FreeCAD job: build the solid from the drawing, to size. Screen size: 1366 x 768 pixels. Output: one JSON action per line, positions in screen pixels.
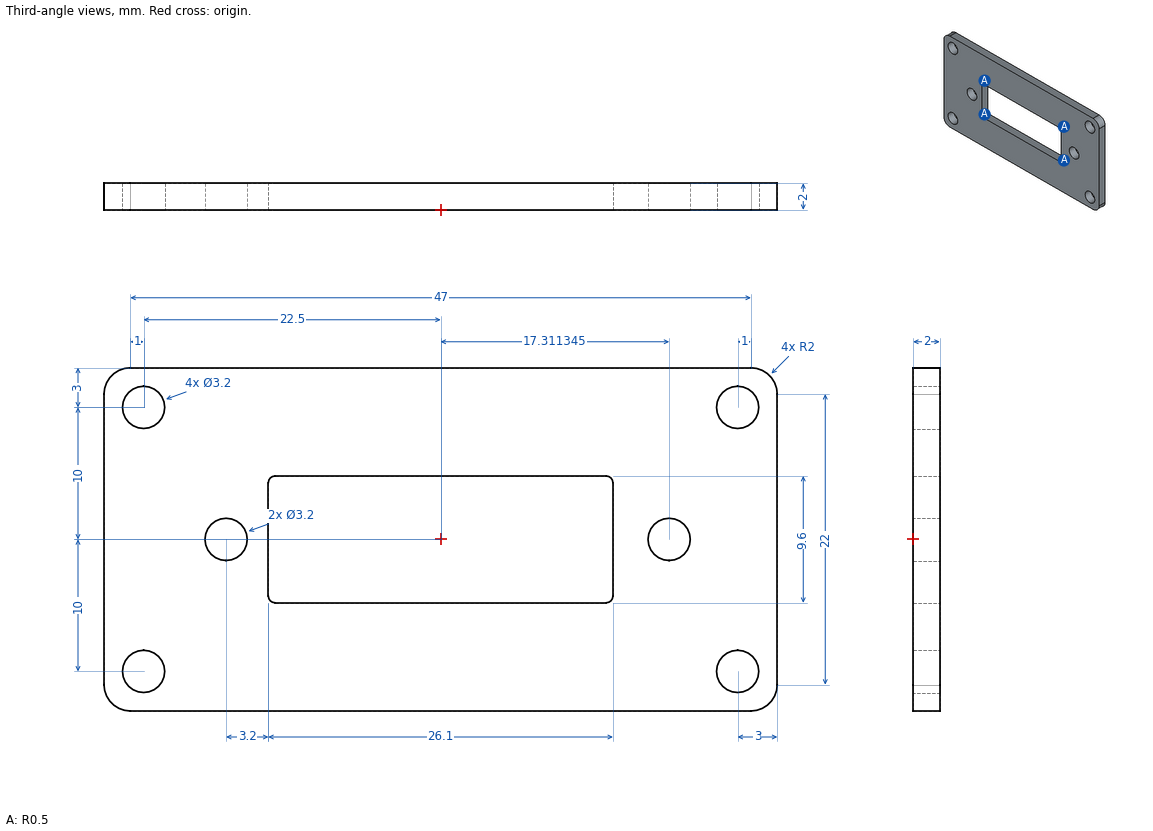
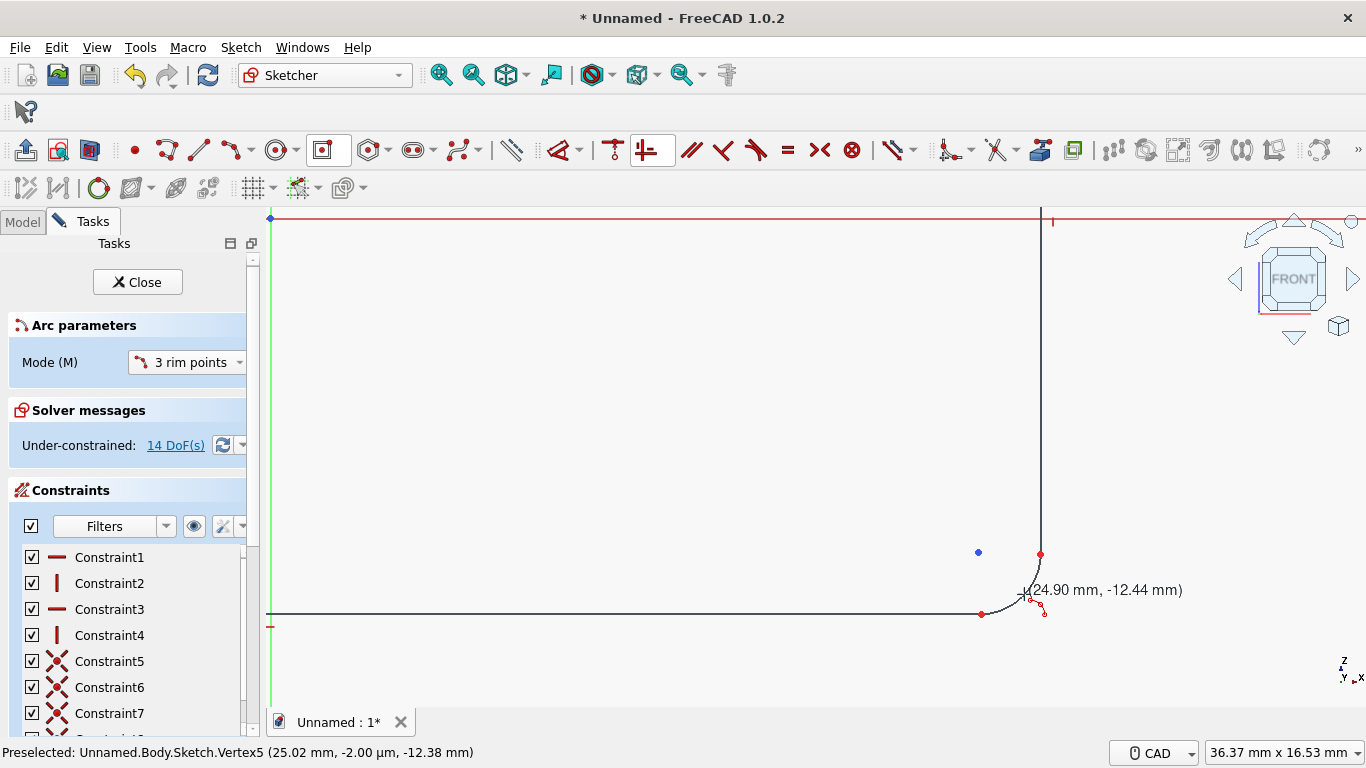
{"action": "scroll", "coordinate": [1025, 596], "scroll_direction": "down", "scroll_amount": 5}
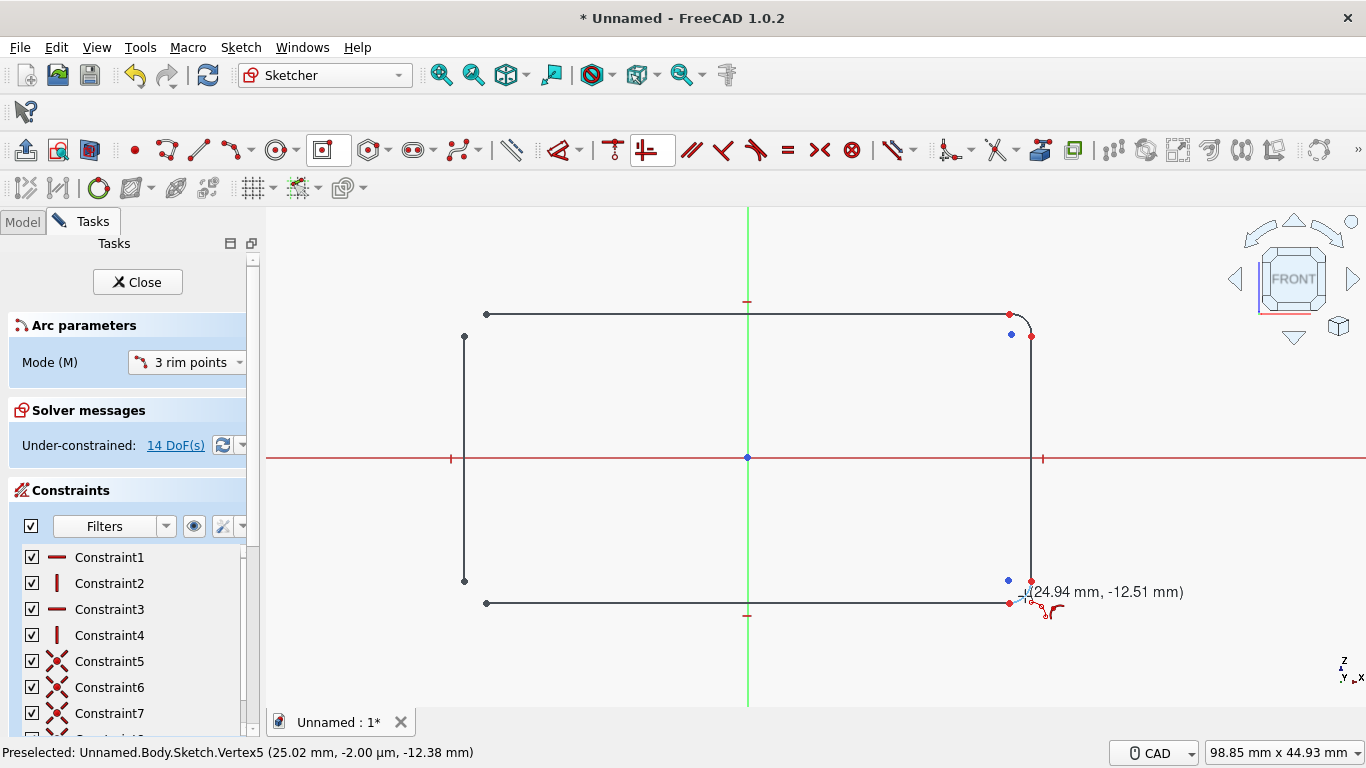
{"action": "left_click", "coordinate": [486, 603]}
{"action": "left_click", "coordinate": [464, 581]}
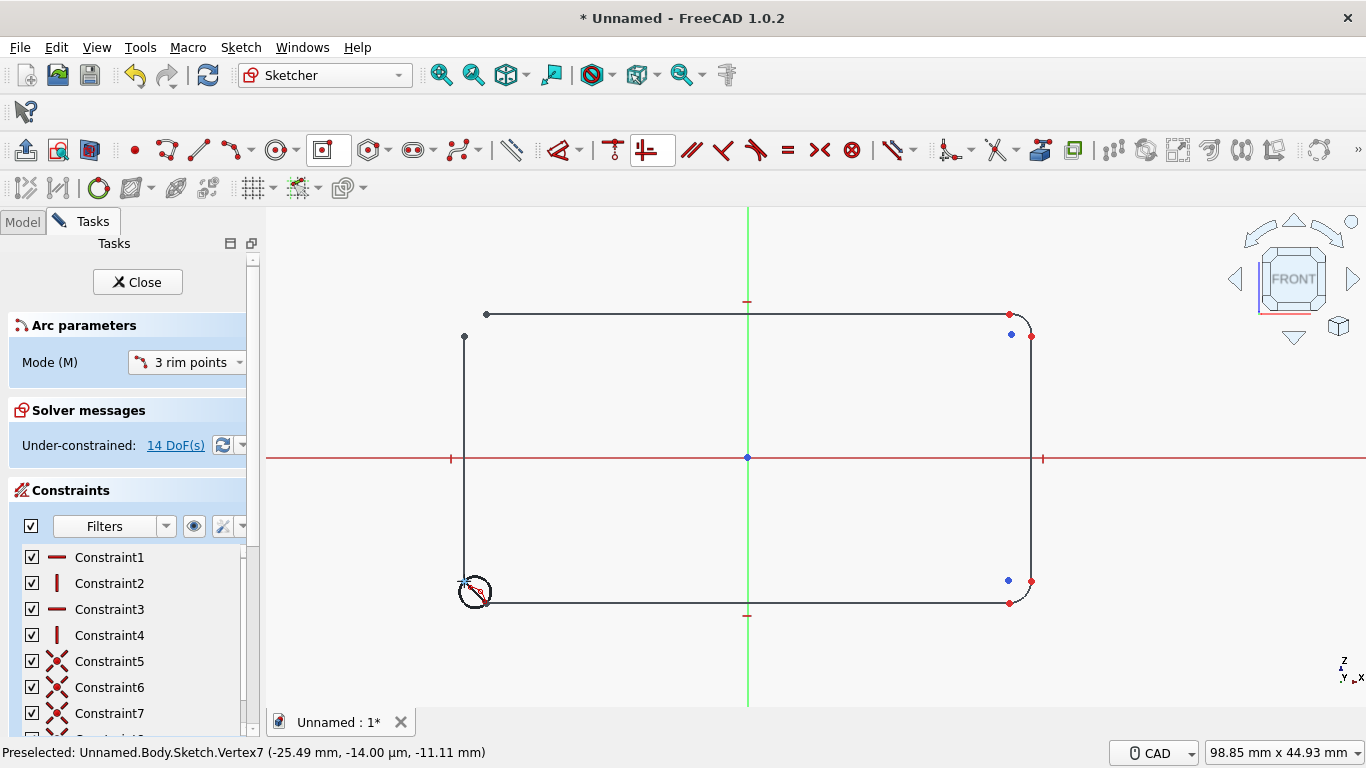
{"action": "scroll", "coordinate": [471, 596], "scroll_direction": "up", "scroll_amount": 5}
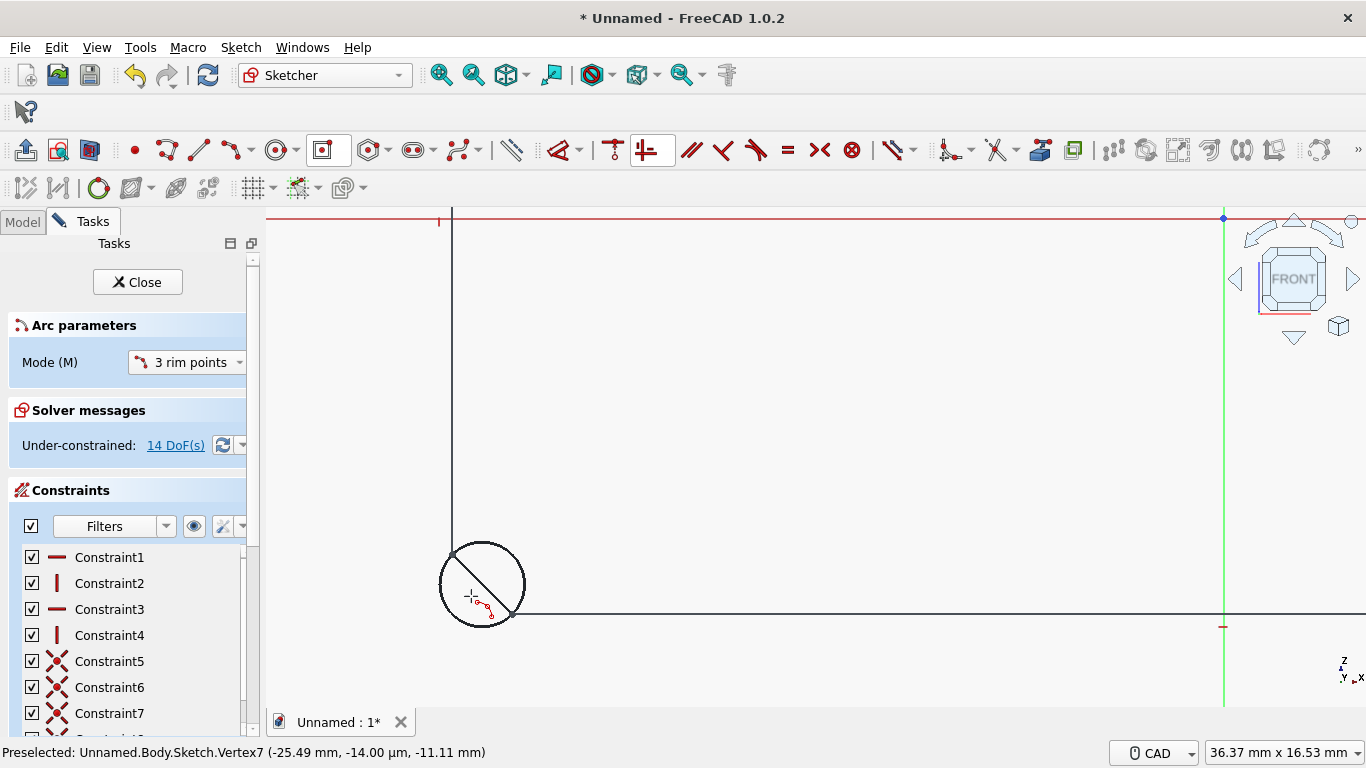
{"action": "left_click", "coordinate": [470, 594]}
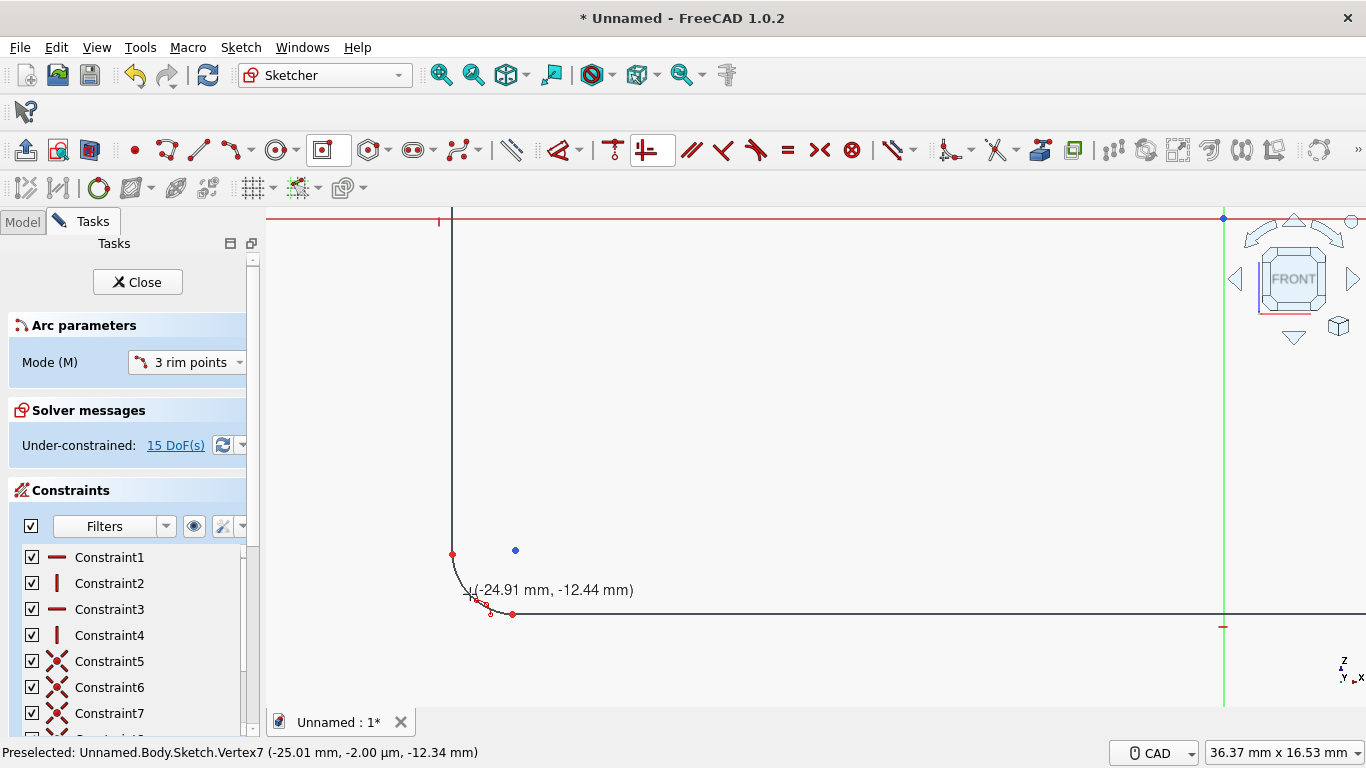
{"action": "scroll", "coordinate": [470, 596], "scroll_direction": "down", "scroll_amount": 5}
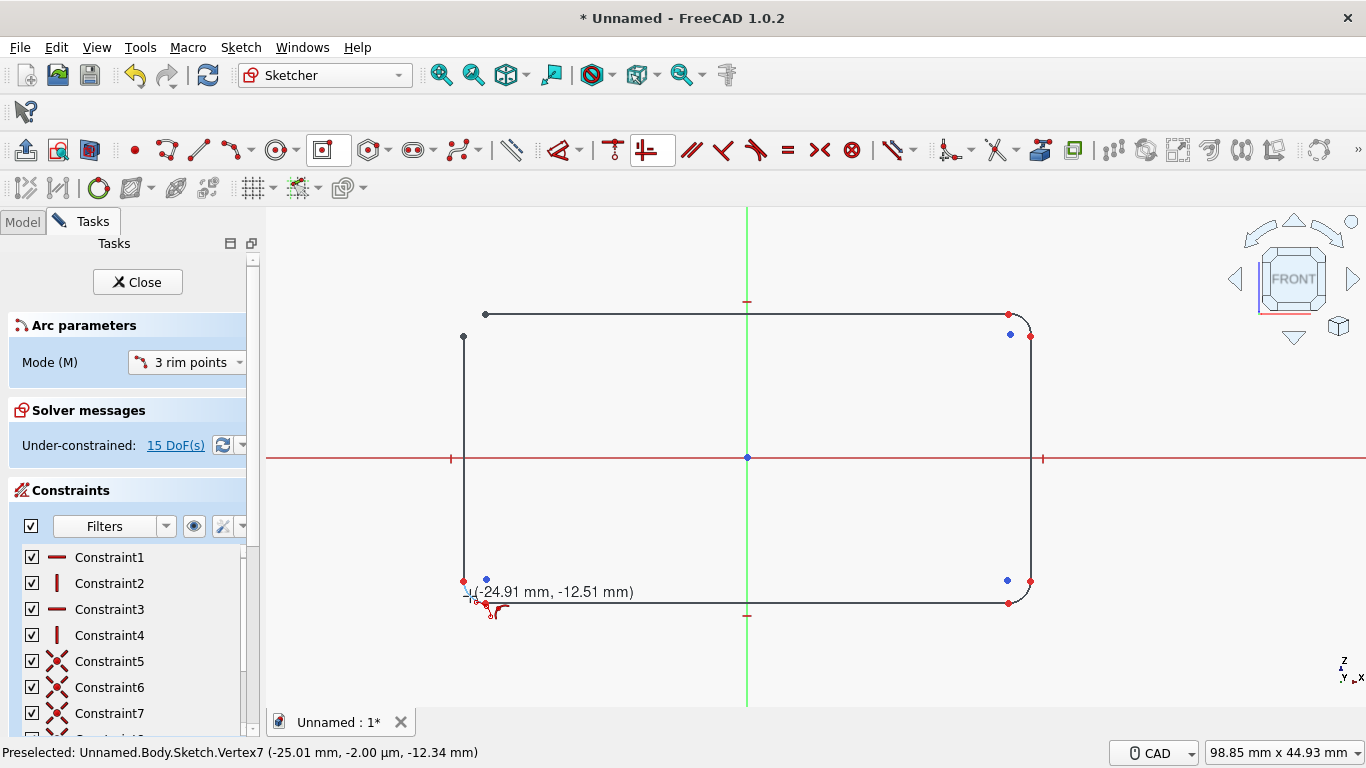
{"action": "left_click", "coordinate": [464, 336]}
{"action": "left_click", "coordinate": [486, 314]}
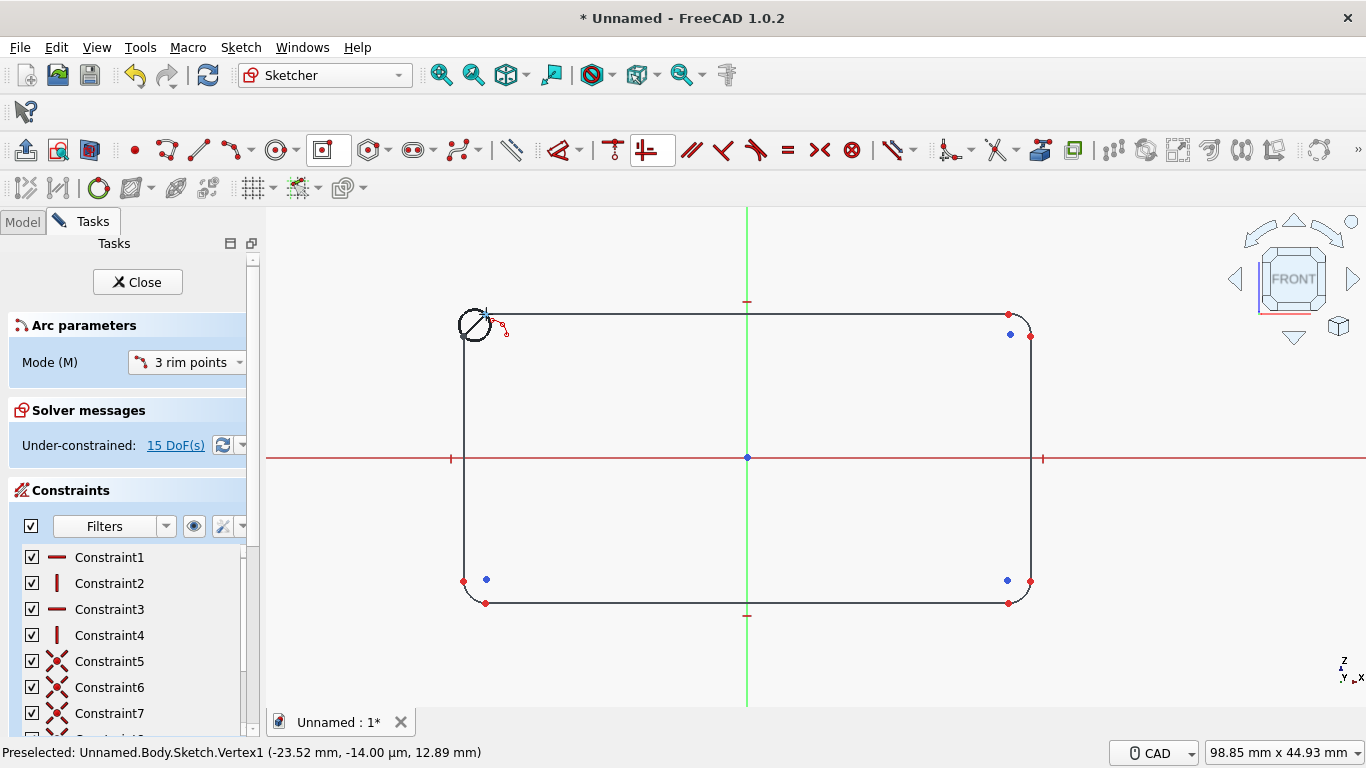
{"action": "scroll", "coordinate": [470, 320], "scroll_direction": "up", "scroll_amount": 5}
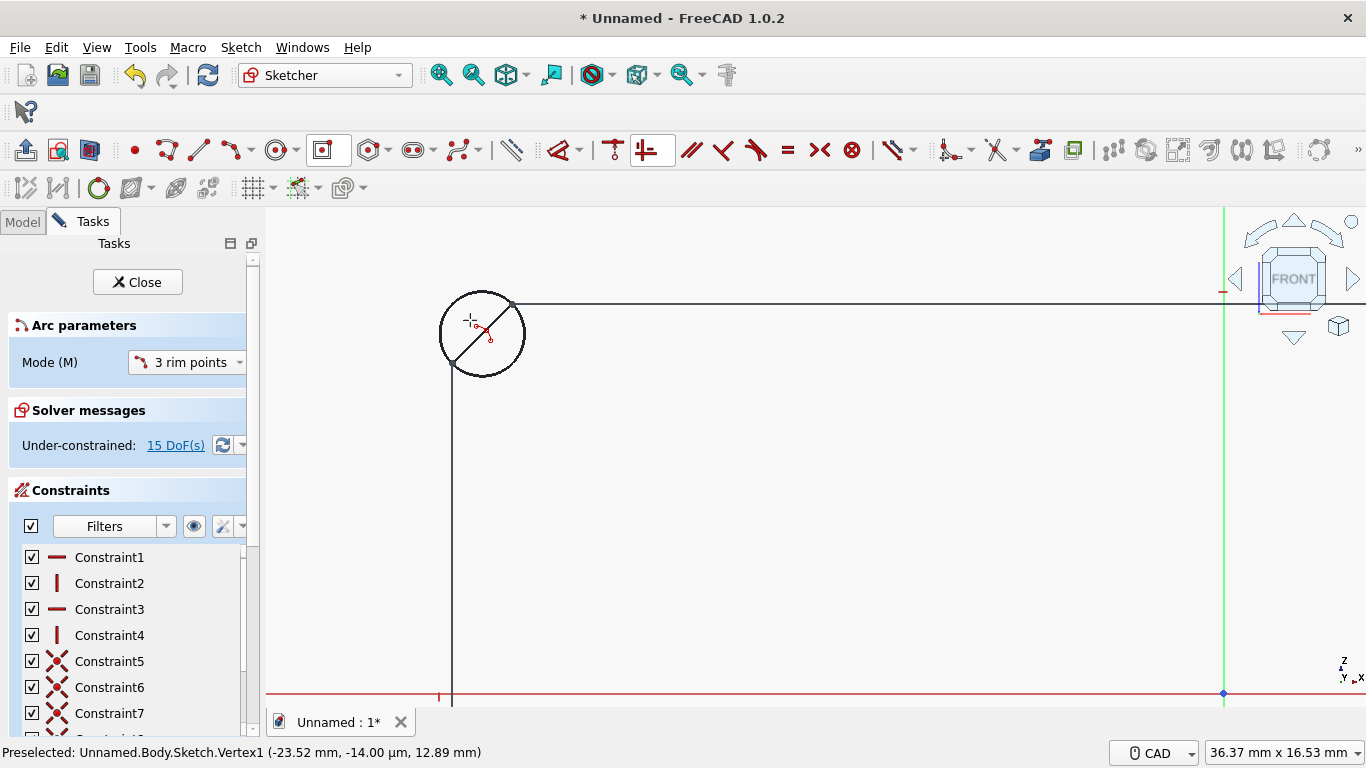
{"action": "left_click", "coordinate": [470, 318]}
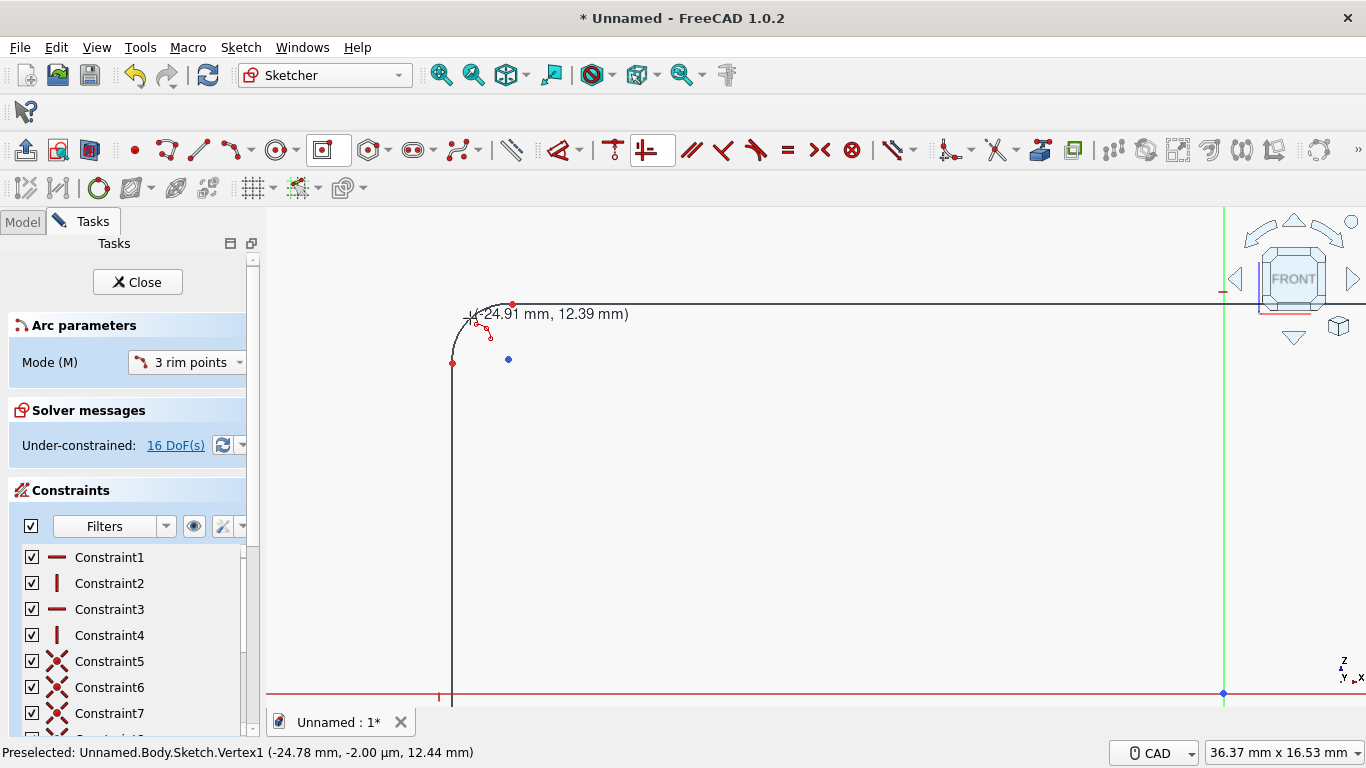
{"action": "left_click", "coordinate": [276, 150]}